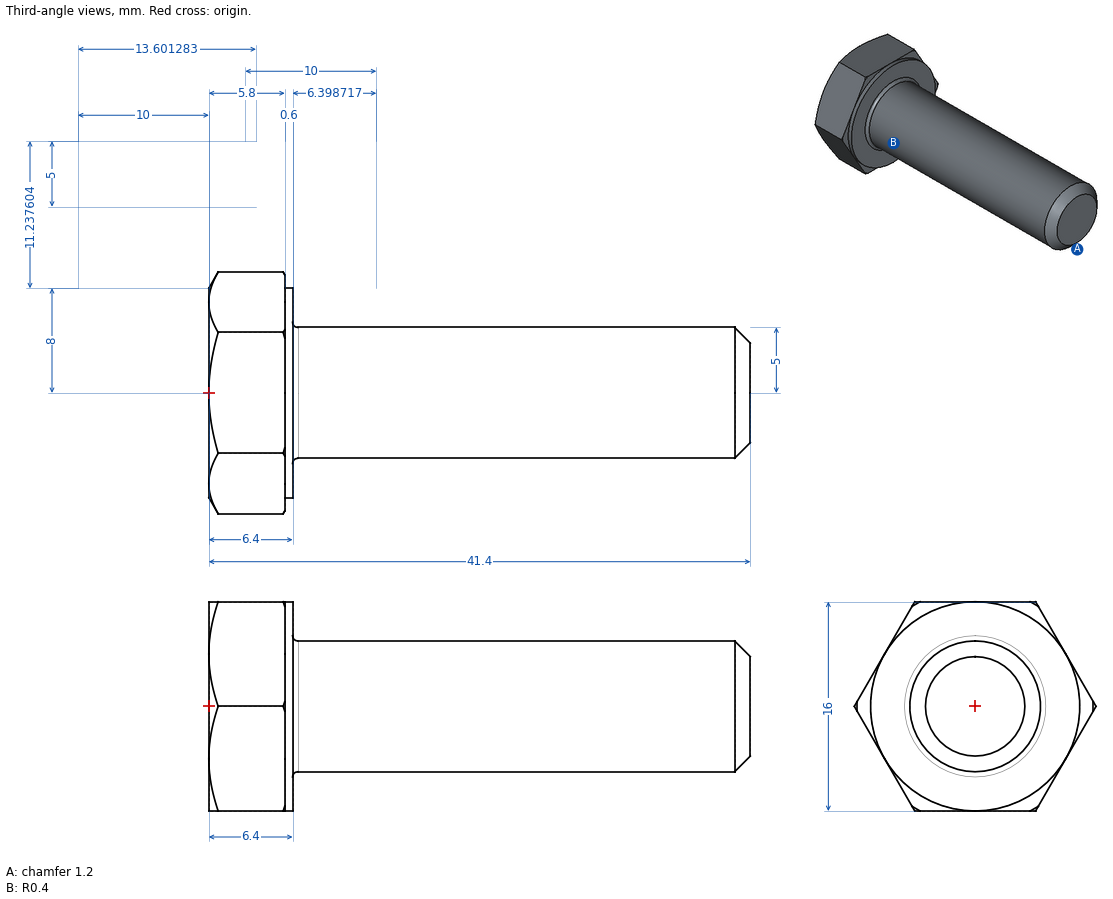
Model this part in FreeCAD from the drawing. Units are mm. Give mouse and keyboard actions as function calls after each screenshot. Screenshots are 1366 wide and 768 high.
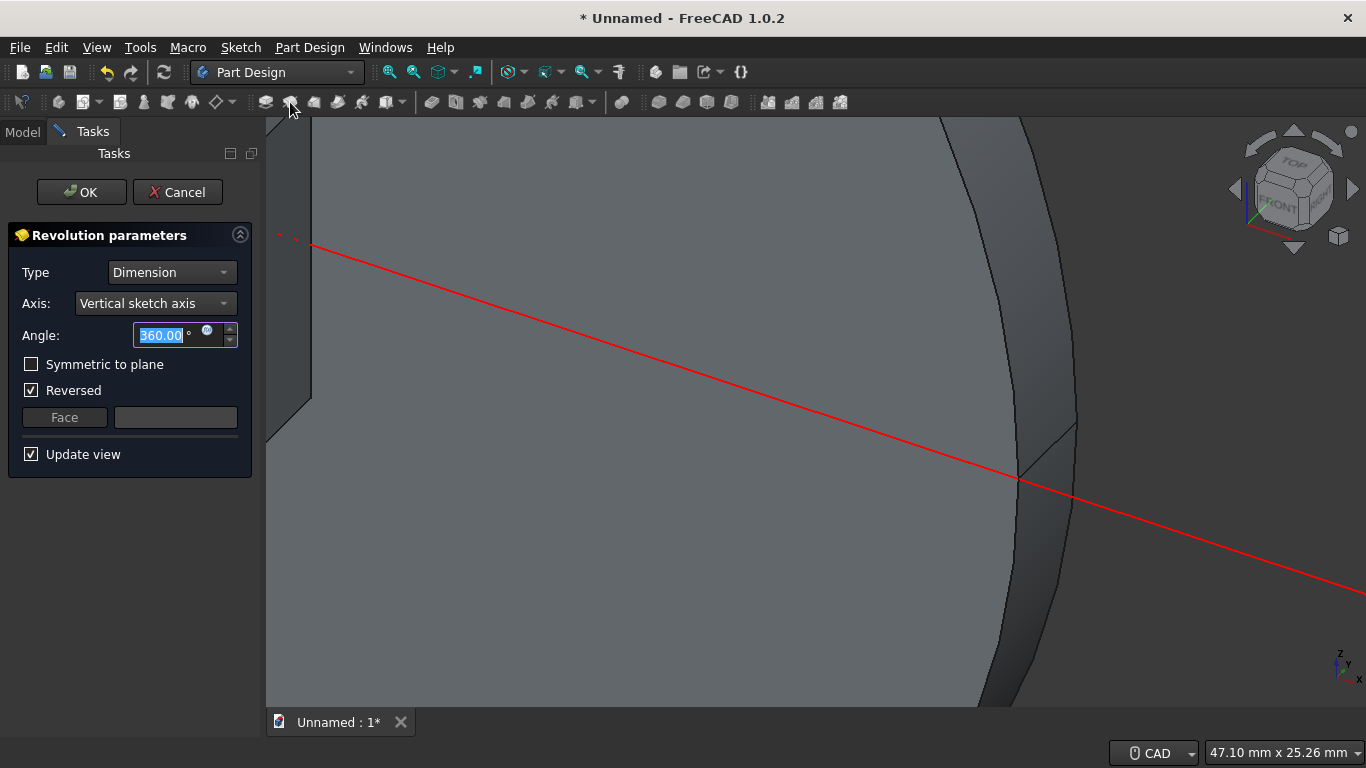
click(156, 304)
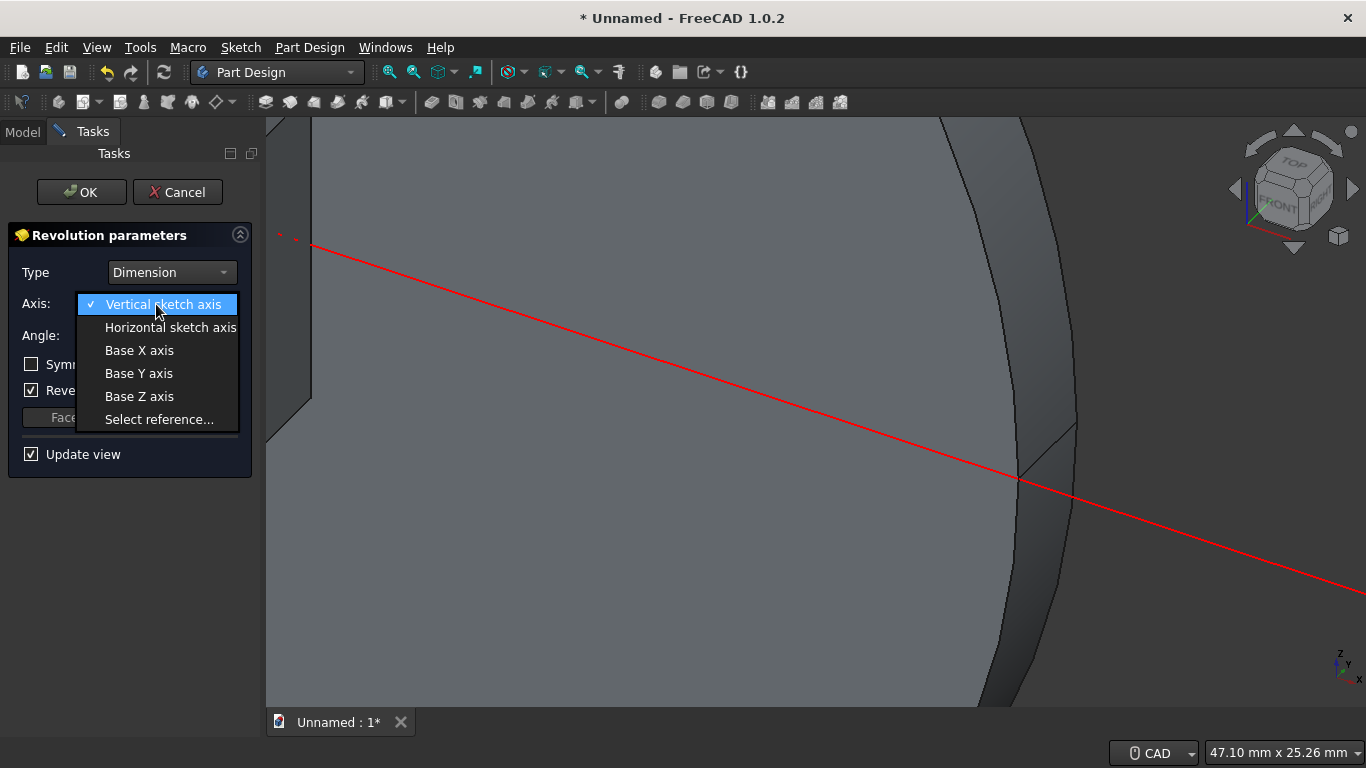
click(156, 328)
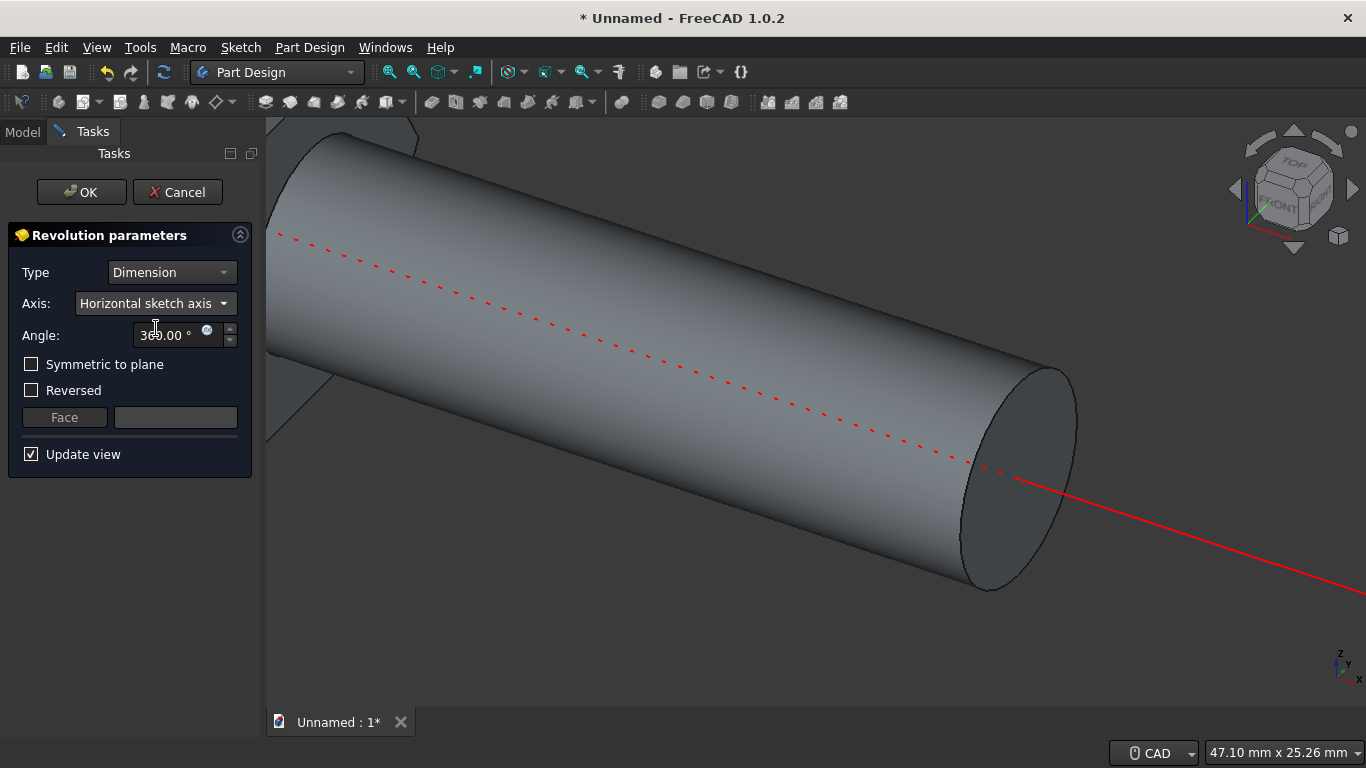
click(82, 192)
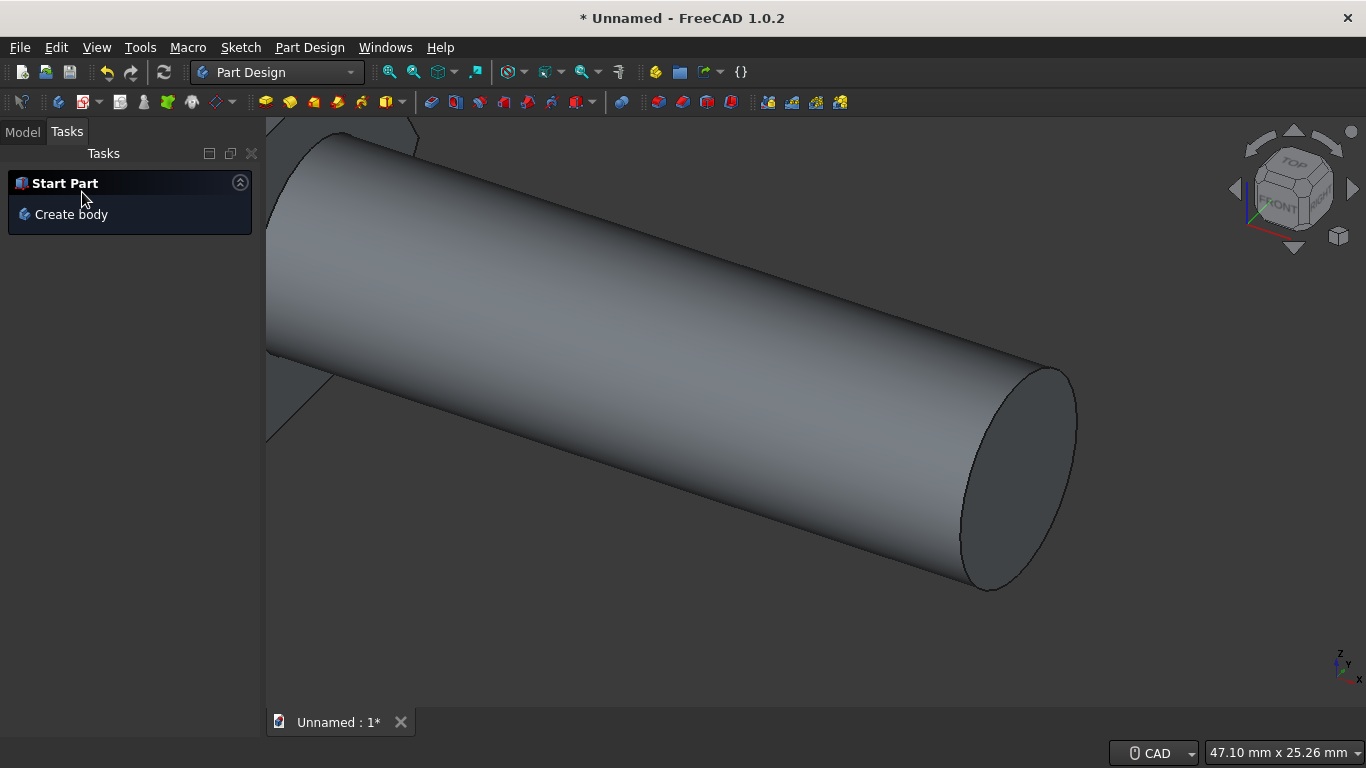
click(390, 72)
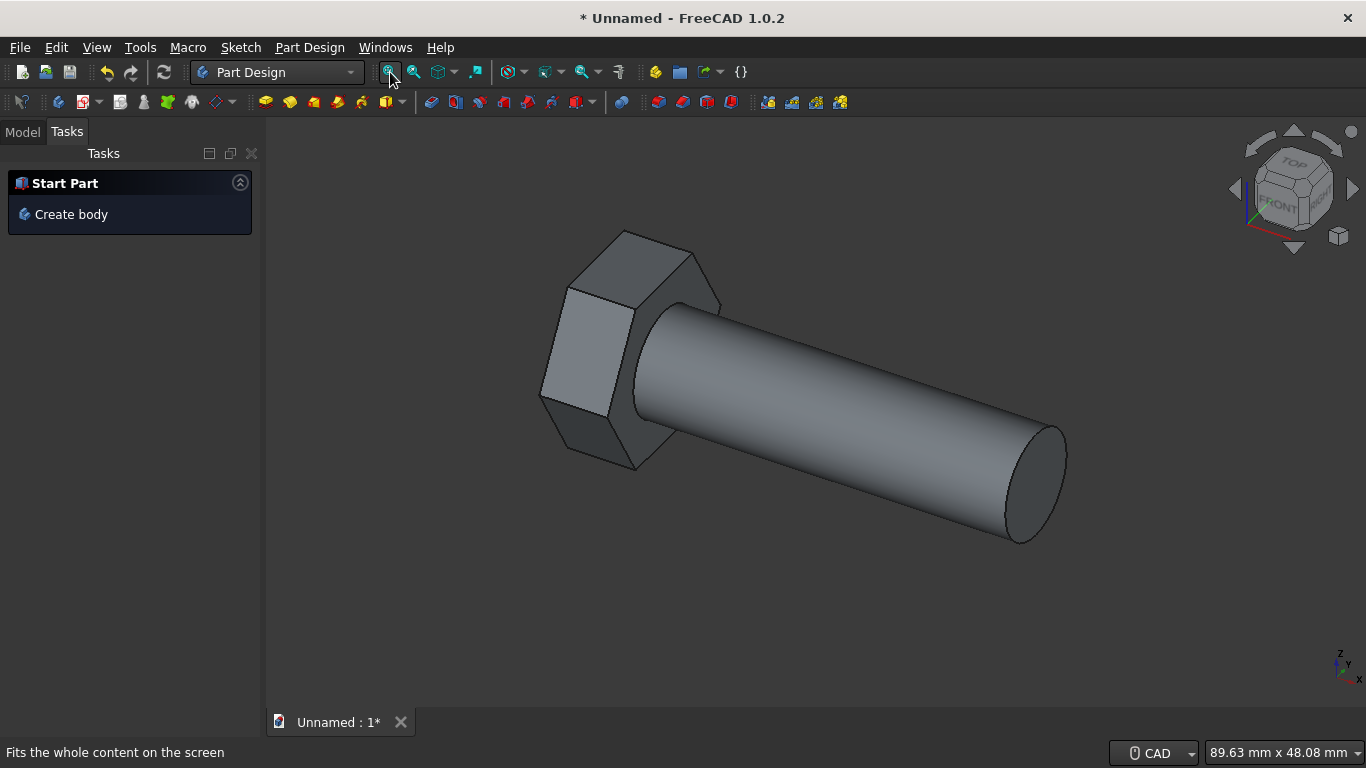
click(84, 102)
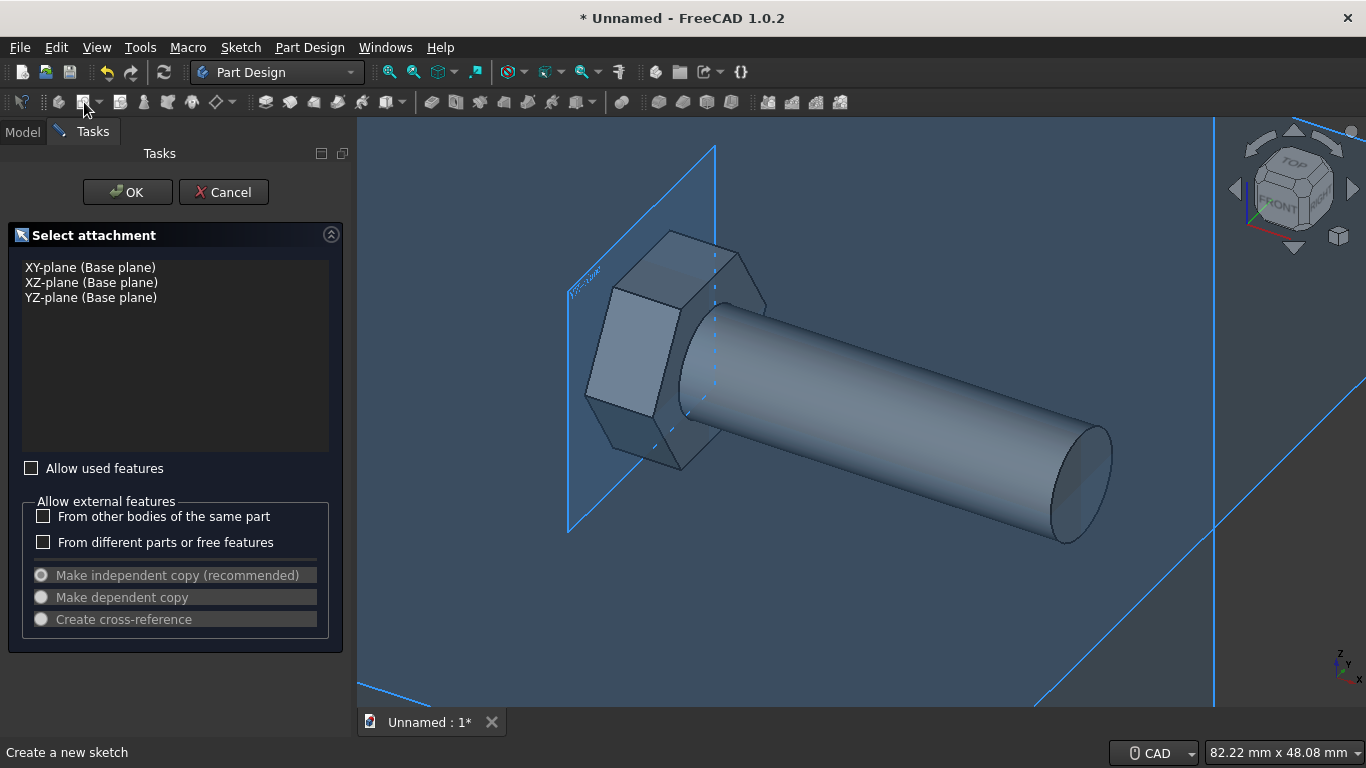
click(82, 268)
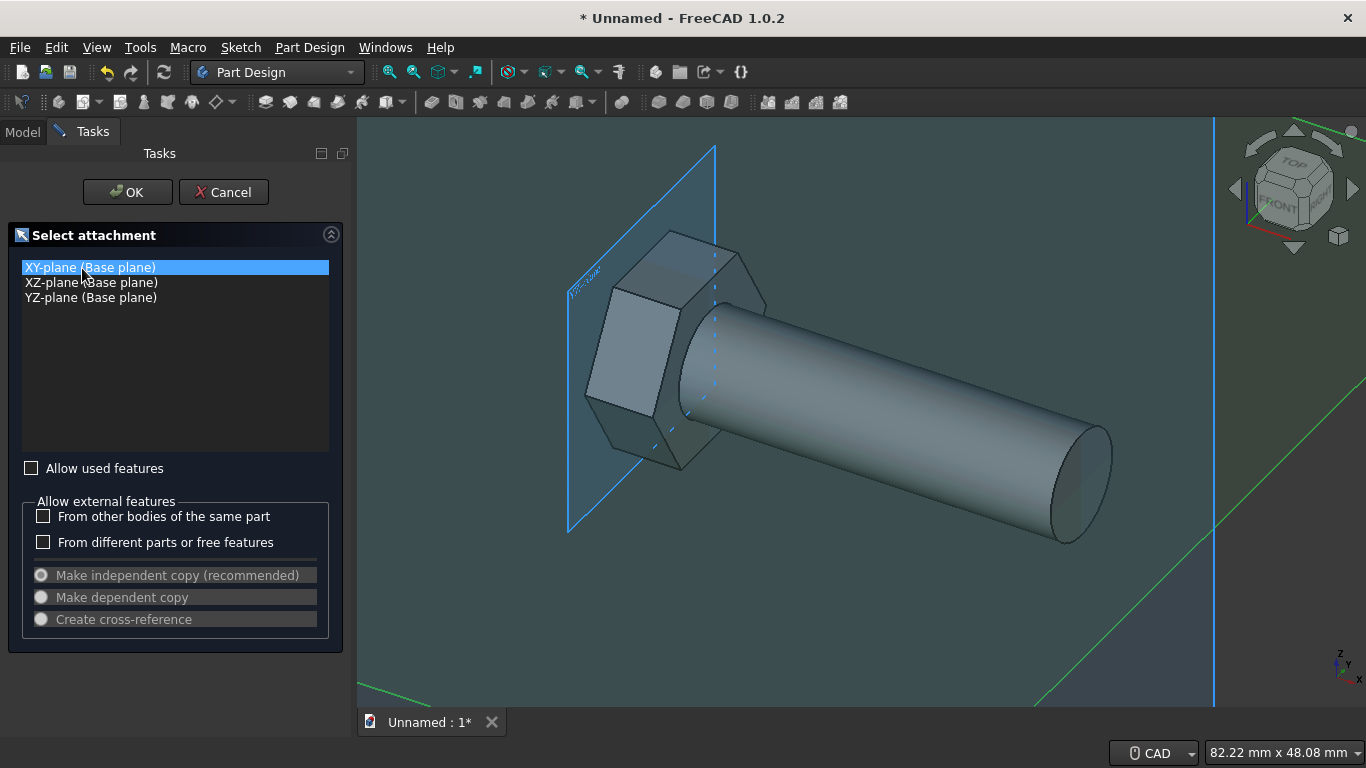
click(128, 192)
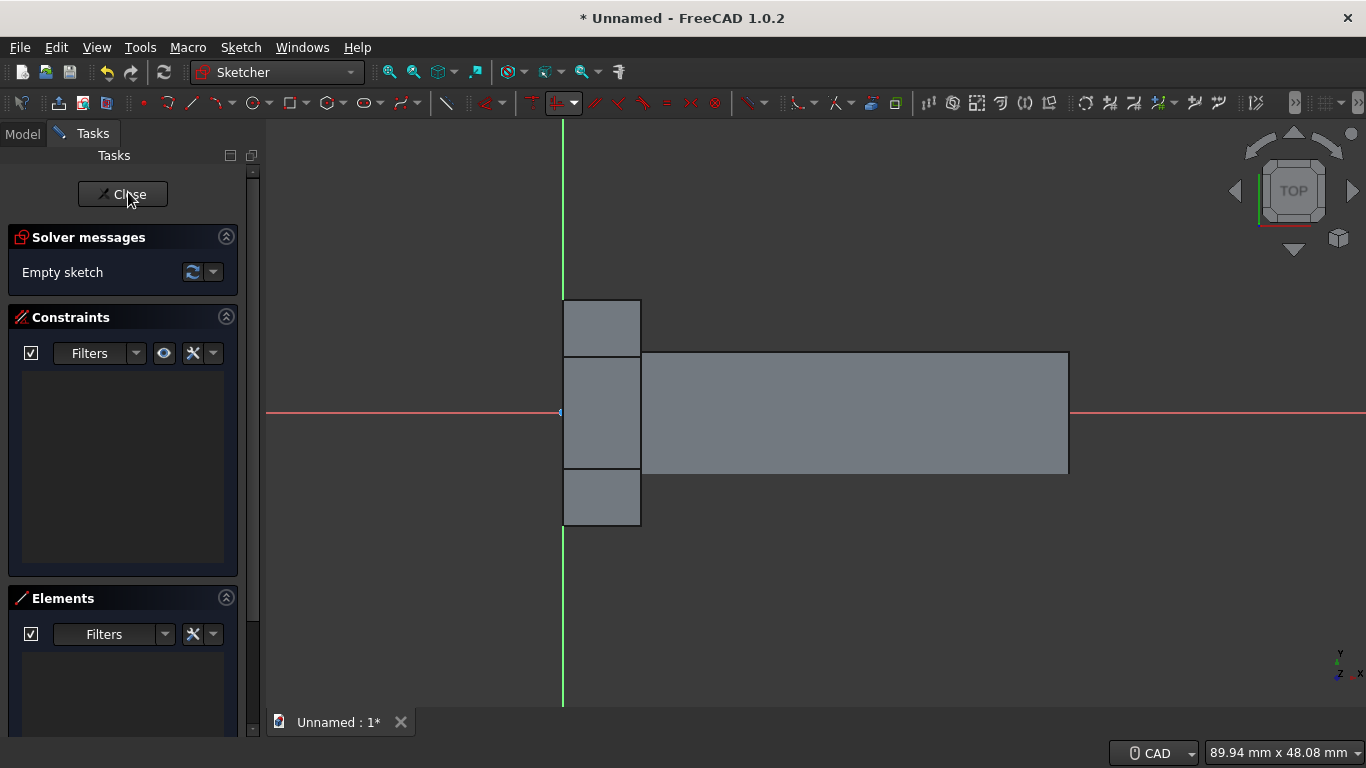
click(108, 104)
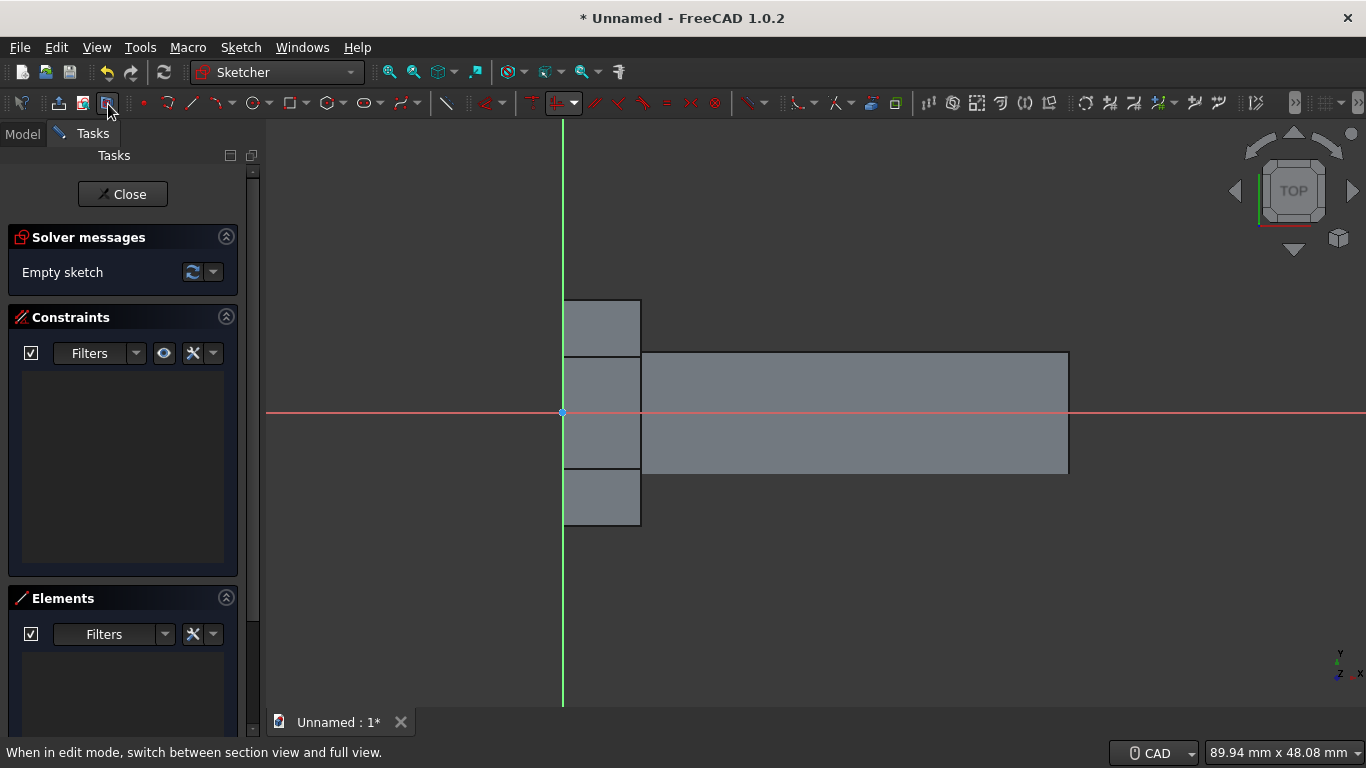
scroll(294, 147, up, 2)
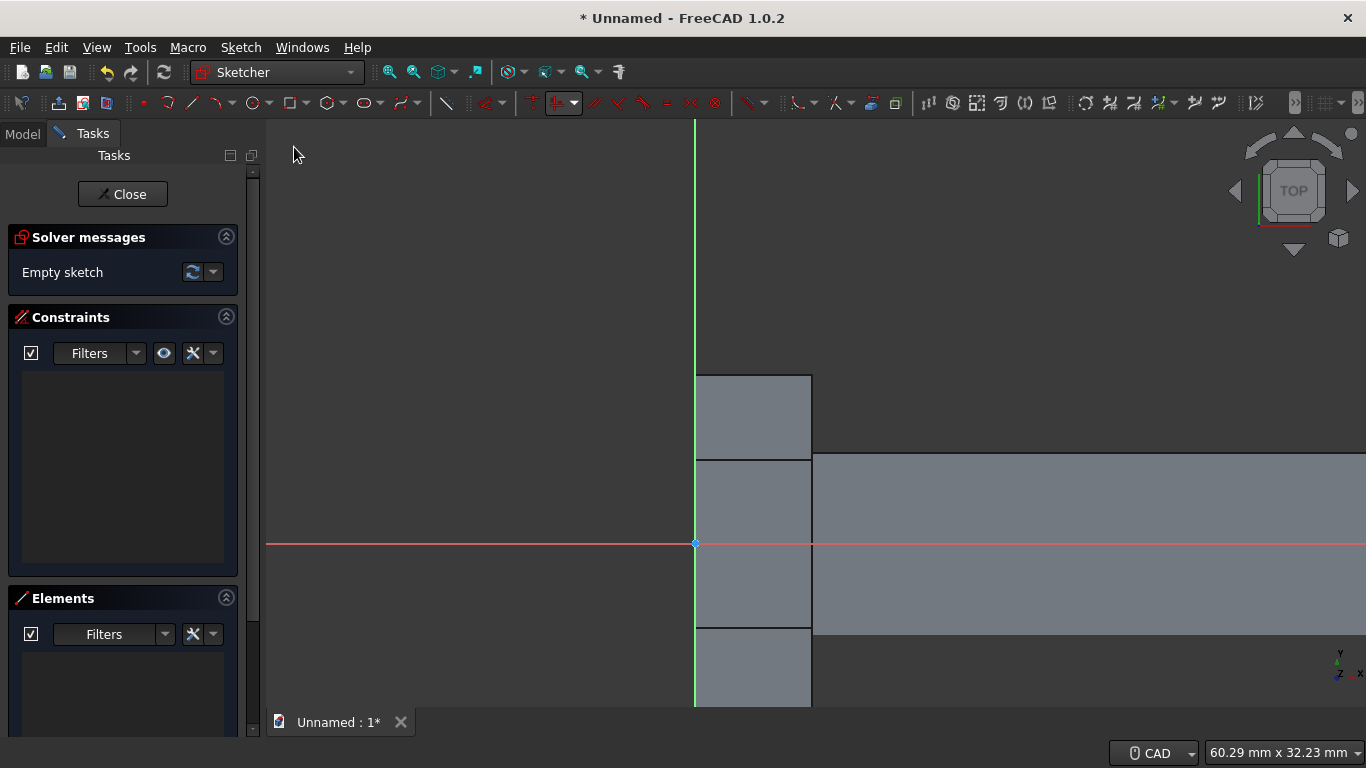
click(168, 104)